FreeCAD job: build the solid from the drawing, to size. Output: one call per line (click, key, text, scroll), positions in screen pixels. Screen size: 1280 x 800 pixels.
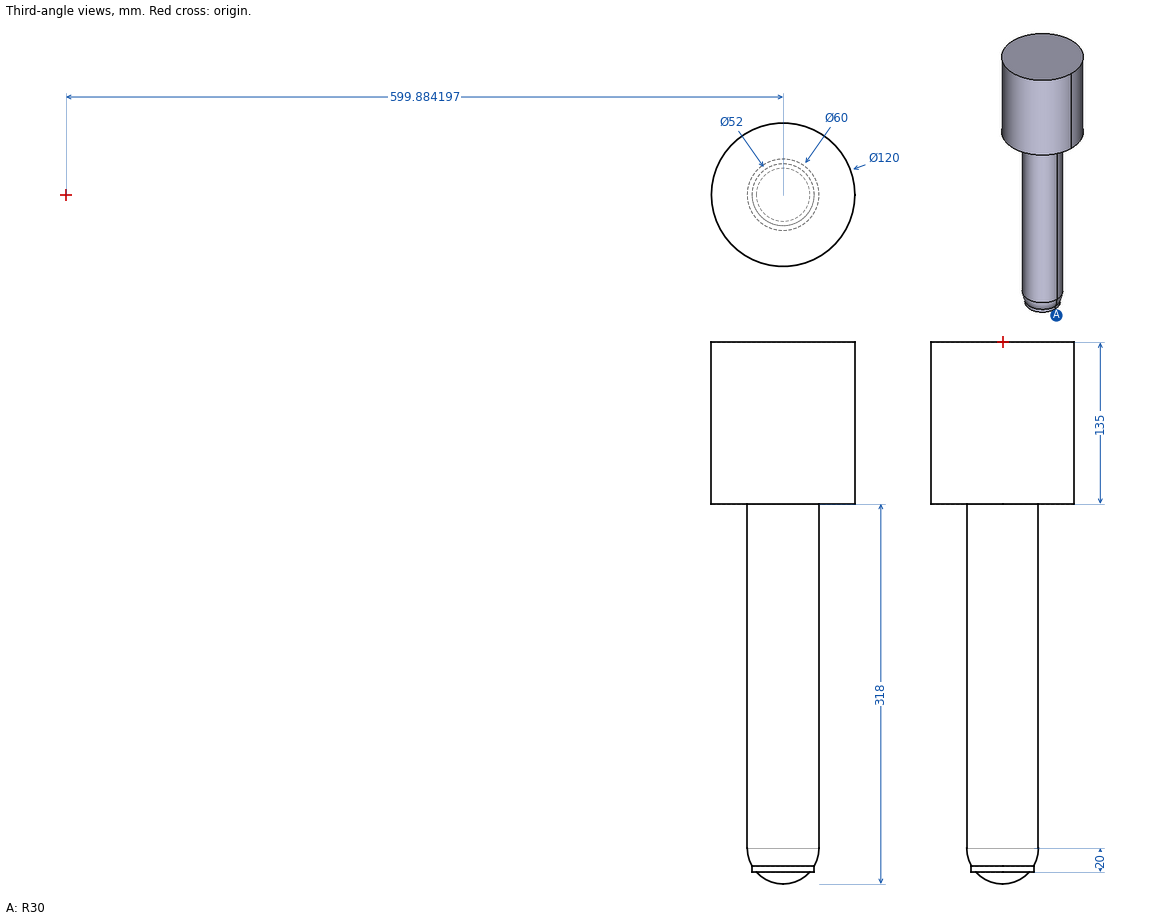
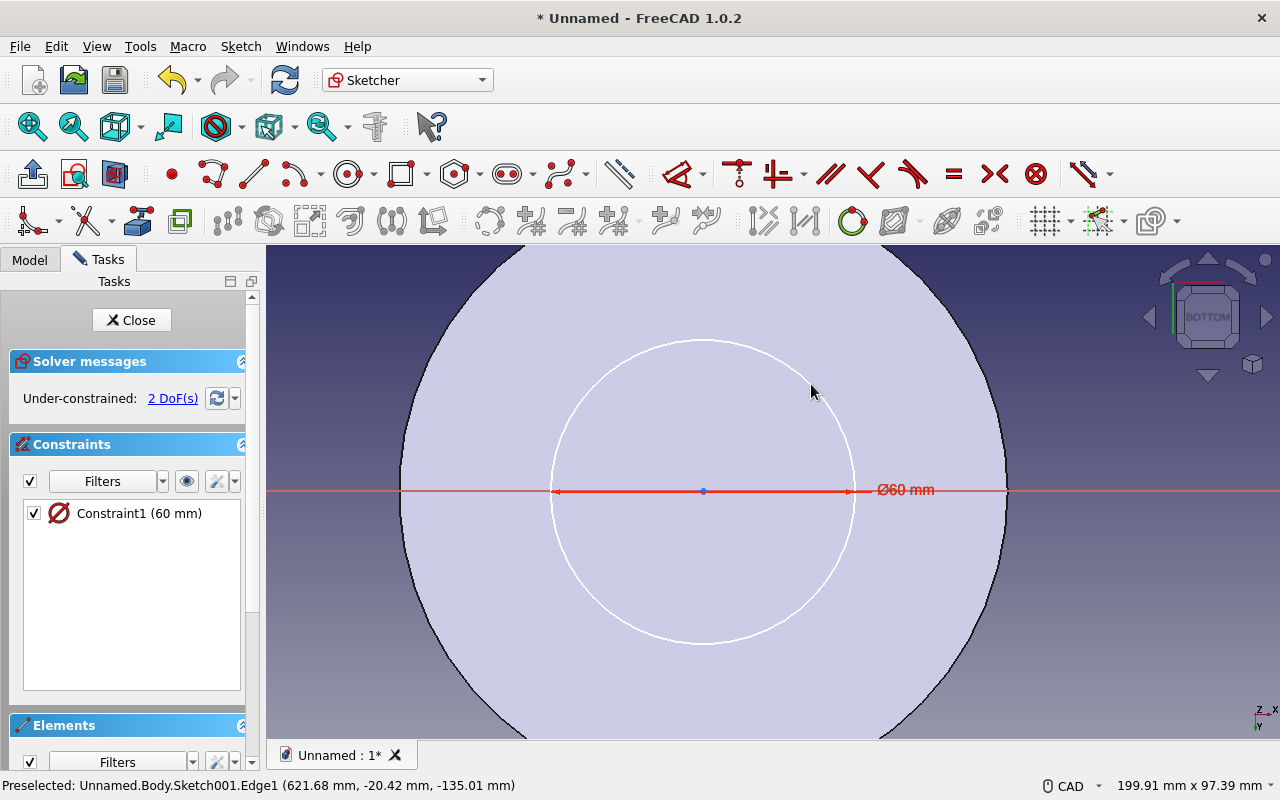
click(703, 492)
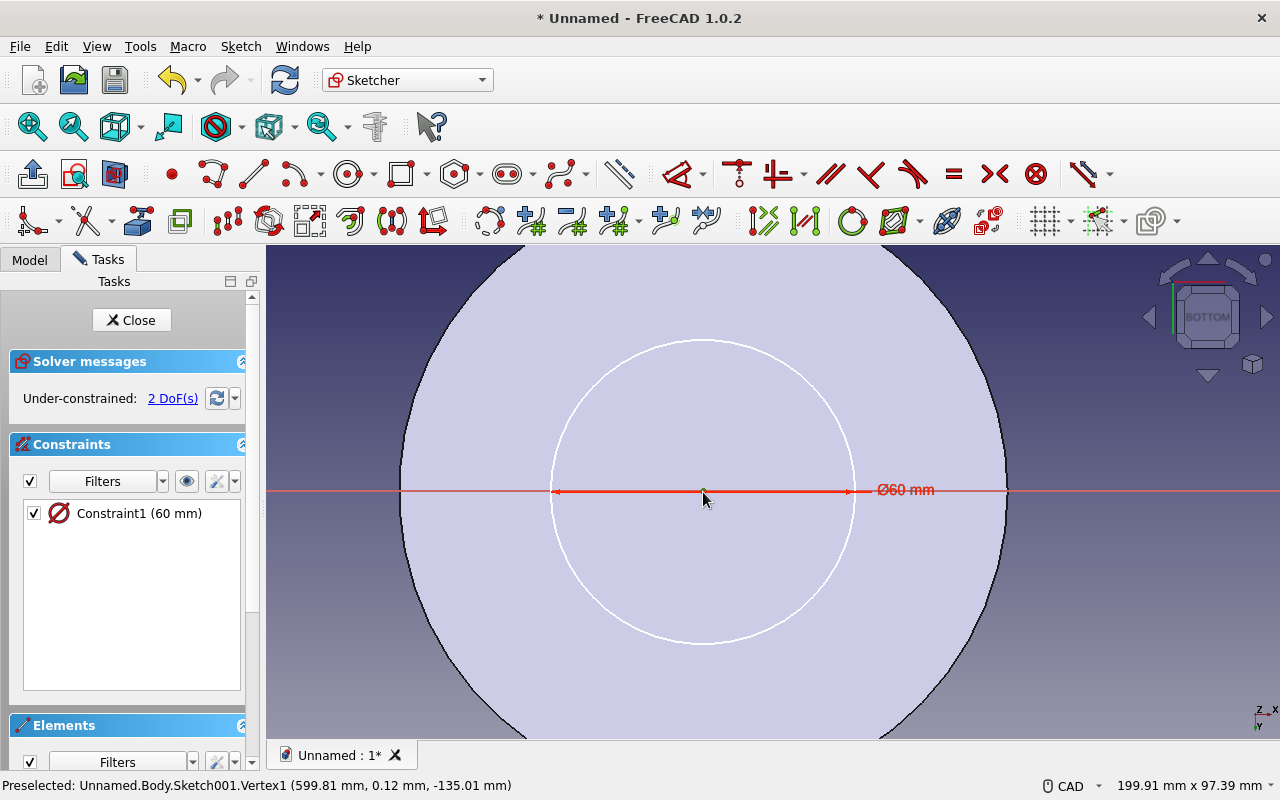
click(353, 491)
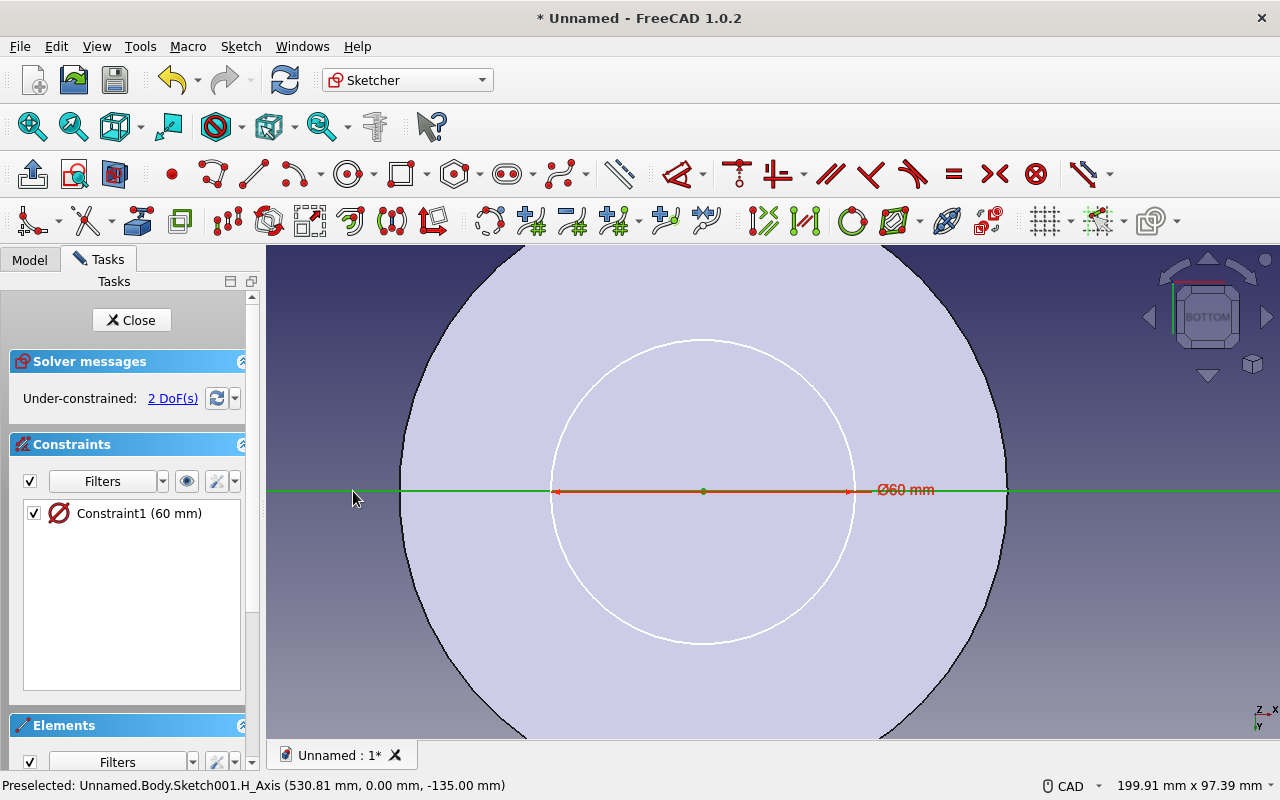
click(737, 174)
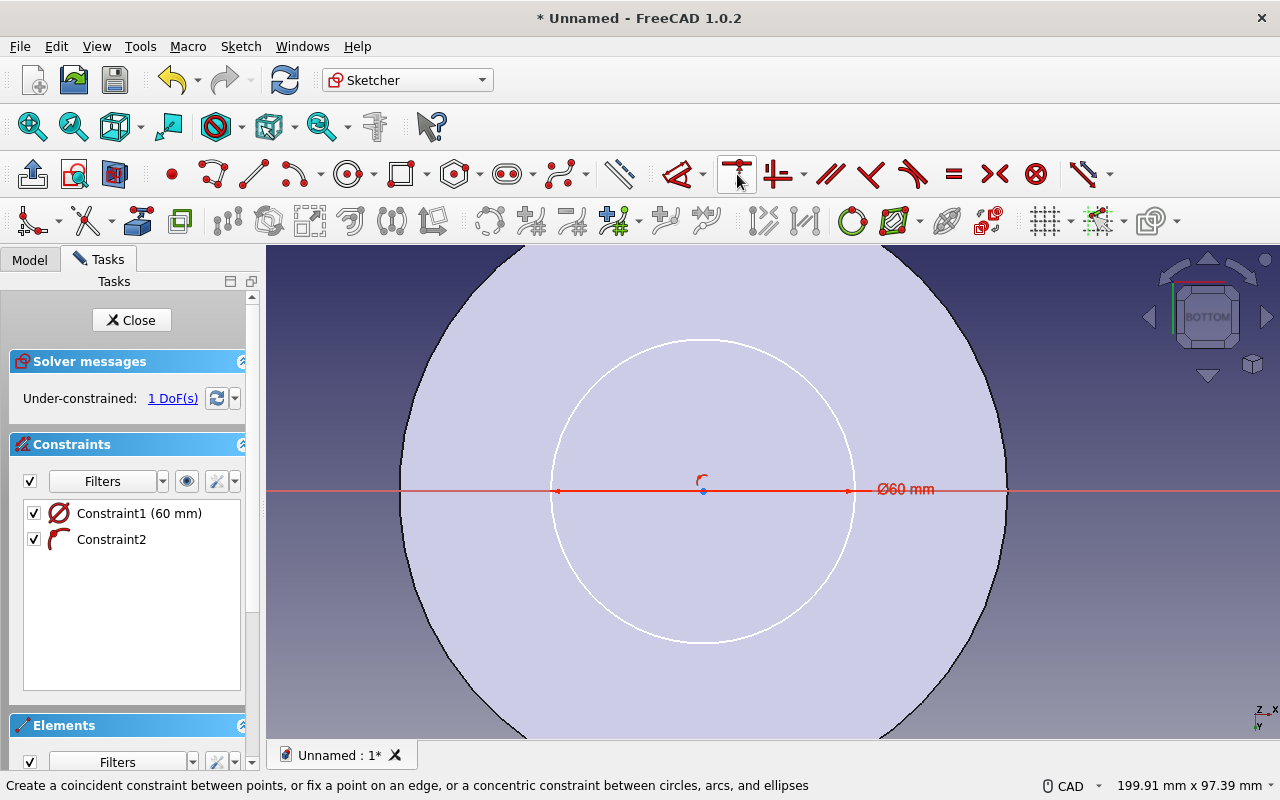
click(676, 174)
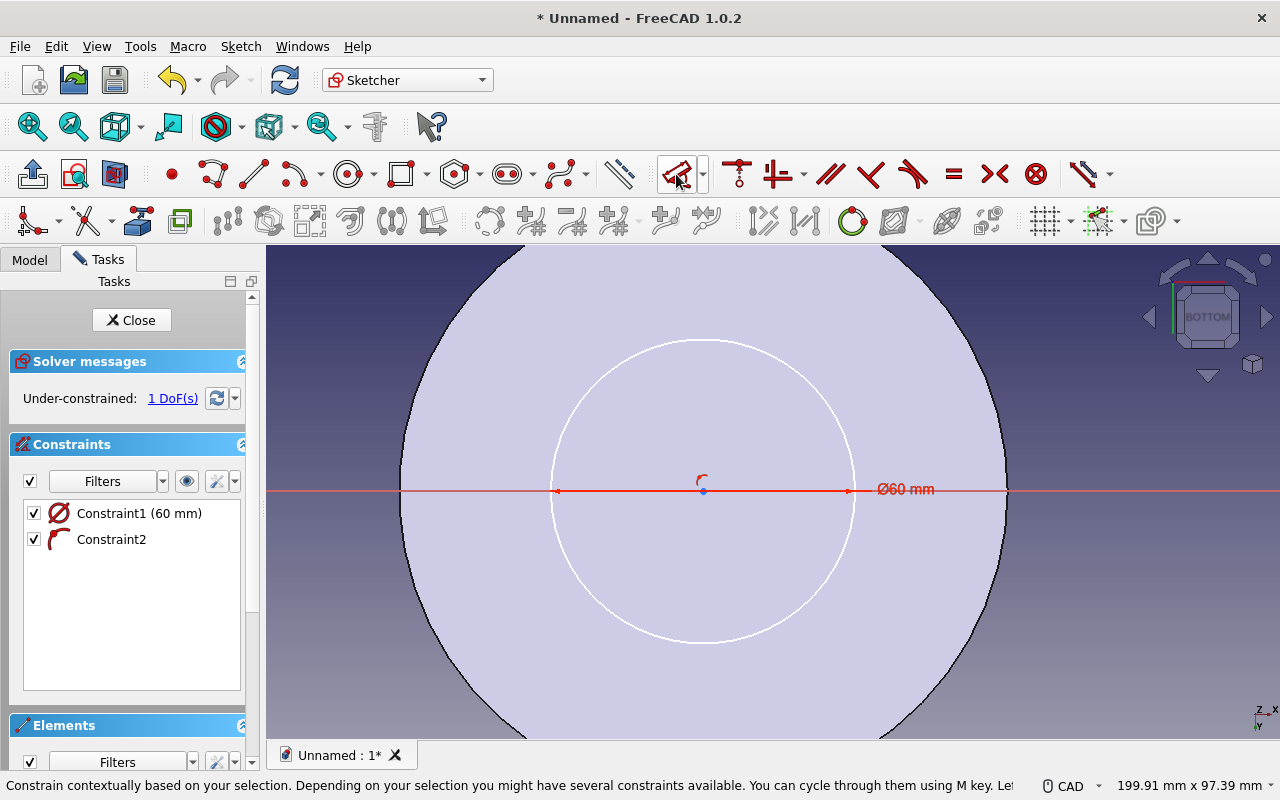
click(703, 491)
click(498, 525)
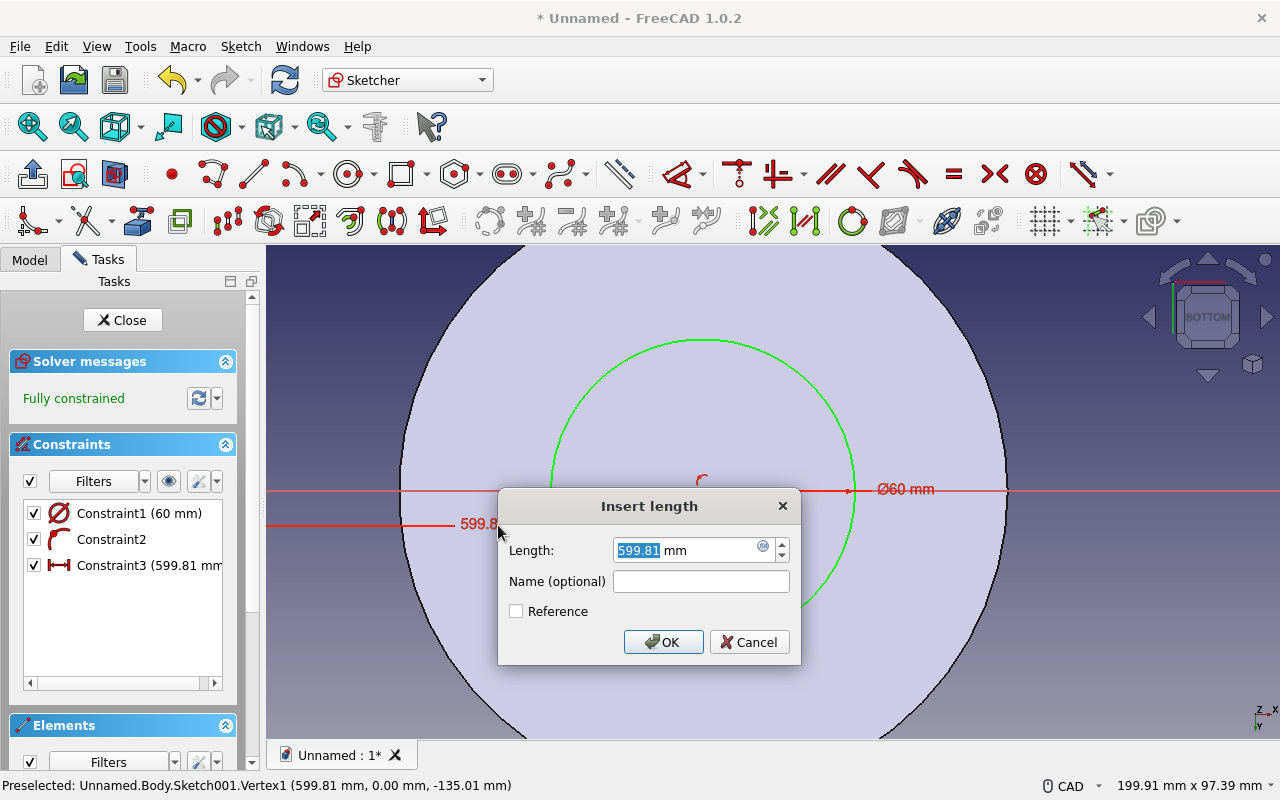
text(599.884197)
key(Return)
key(Escape)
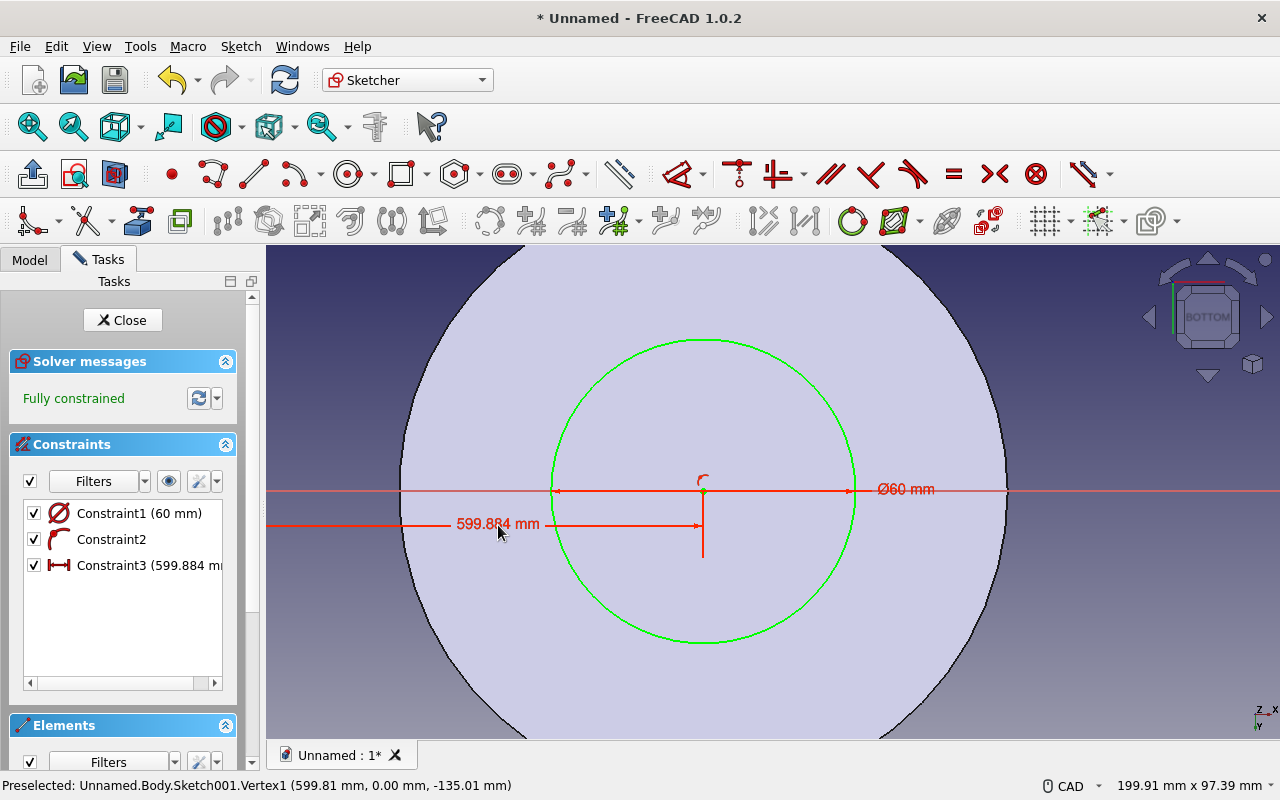
click(123, 320)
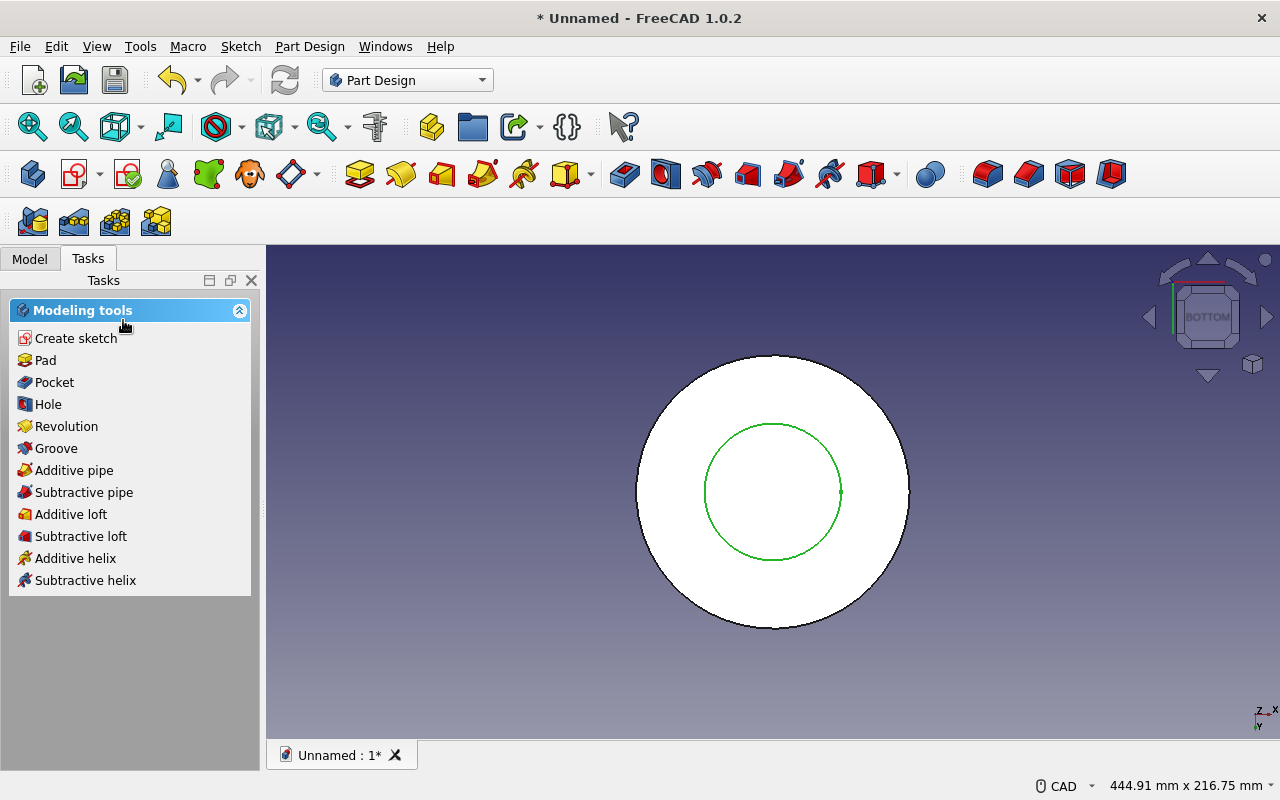
click(360, 174)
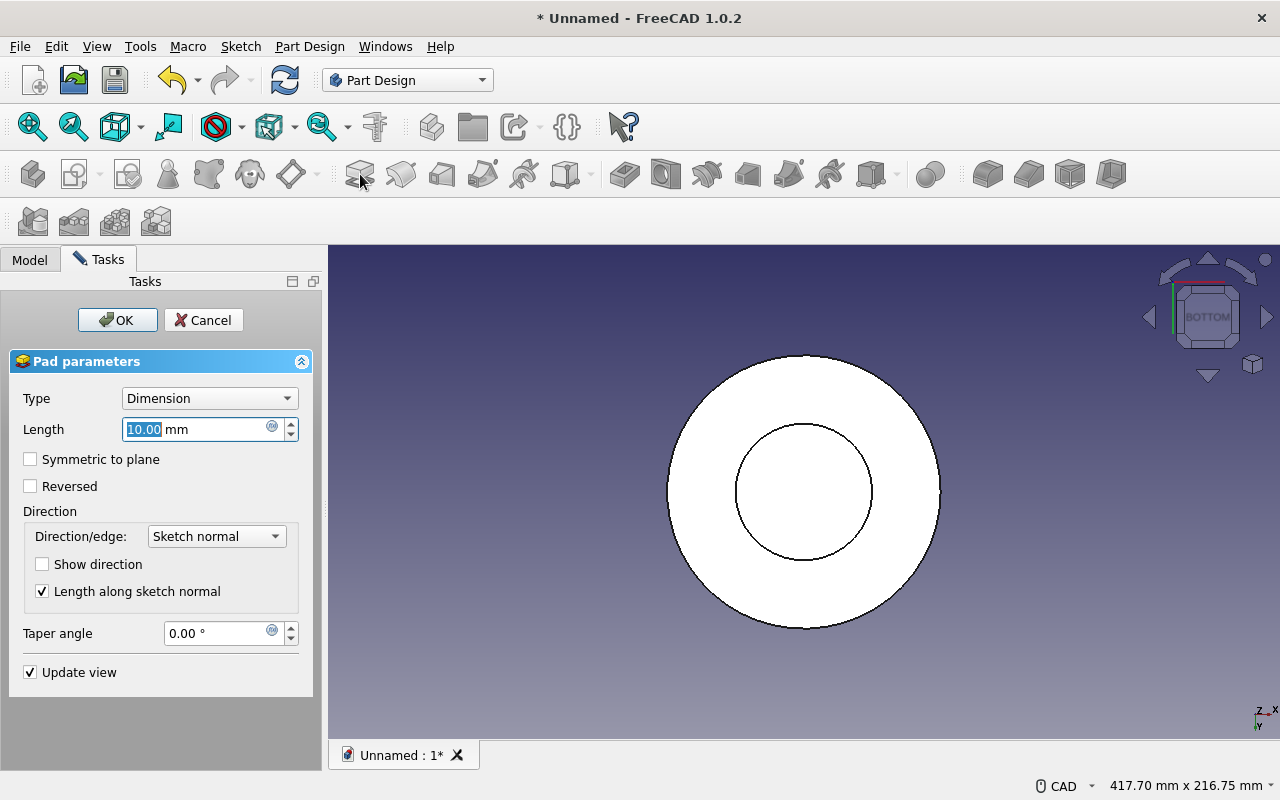
text(318)
key(Tab)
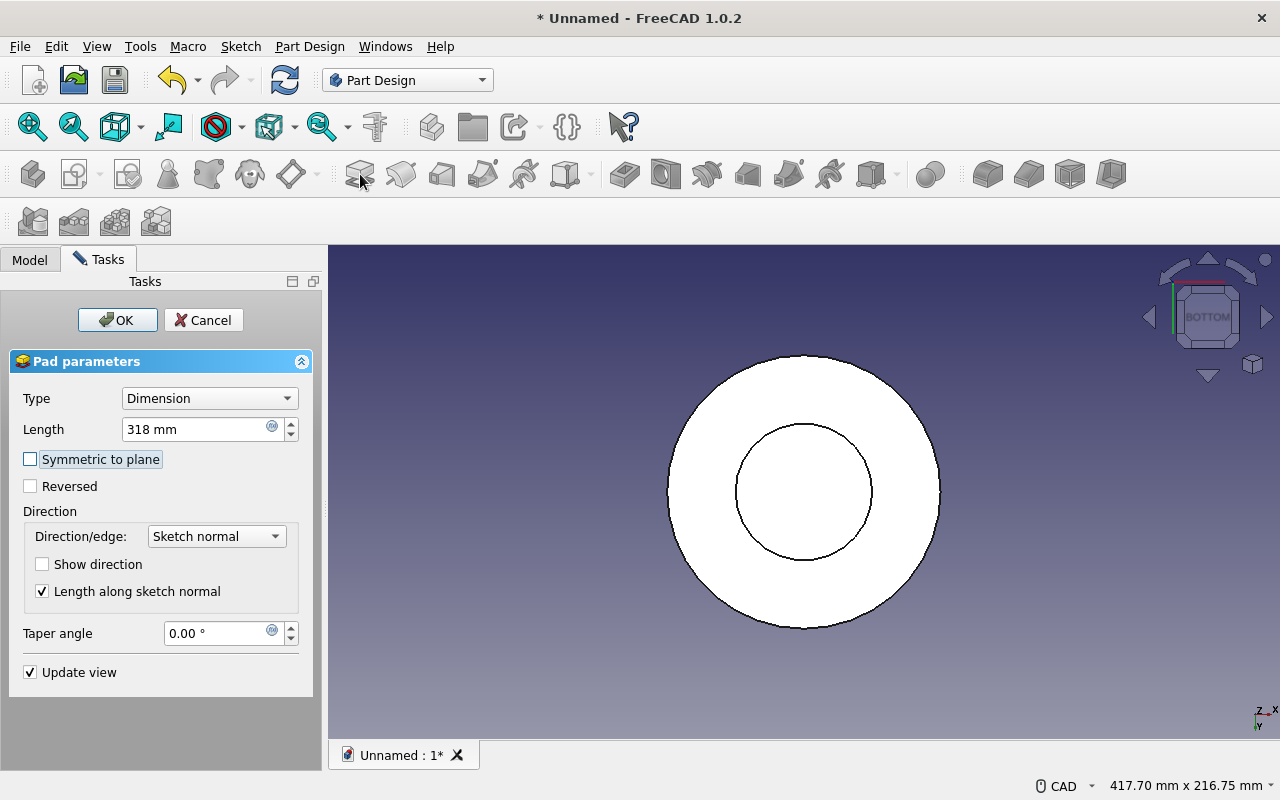
click(118, 320)